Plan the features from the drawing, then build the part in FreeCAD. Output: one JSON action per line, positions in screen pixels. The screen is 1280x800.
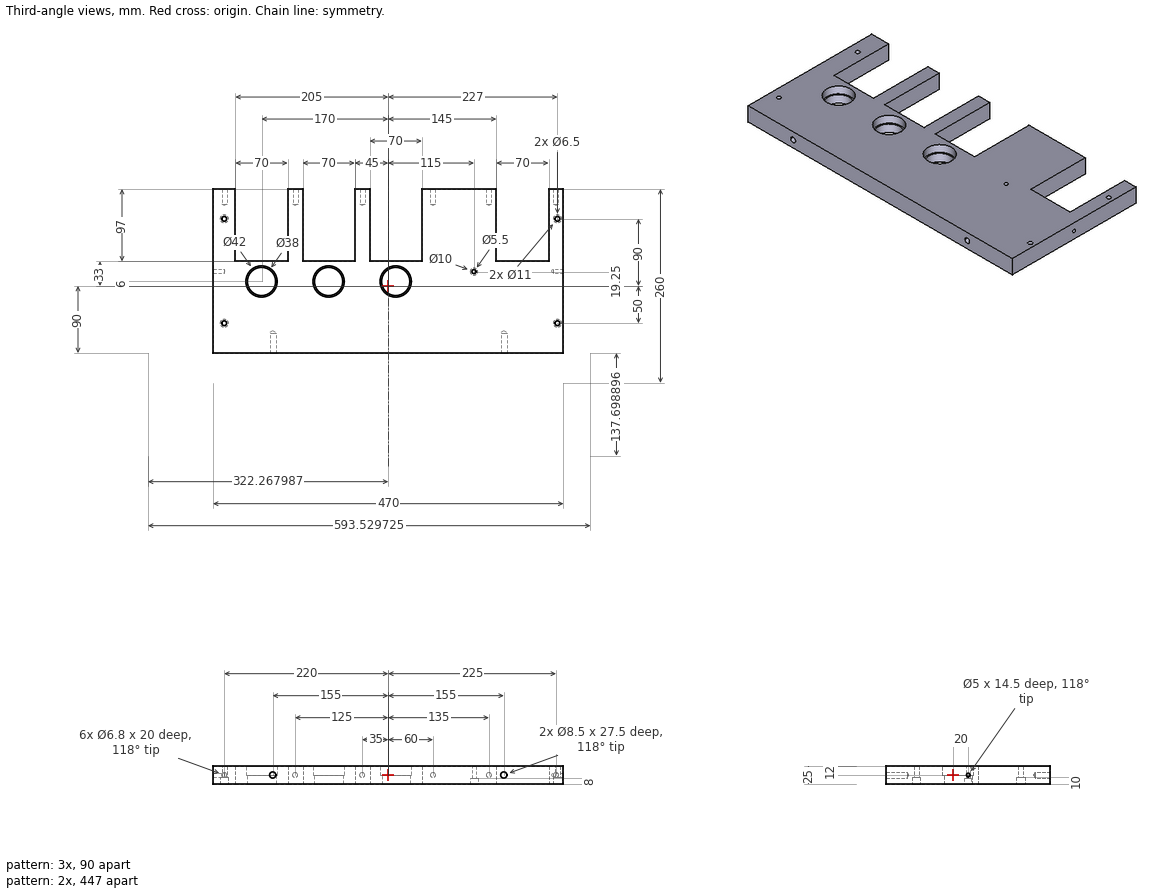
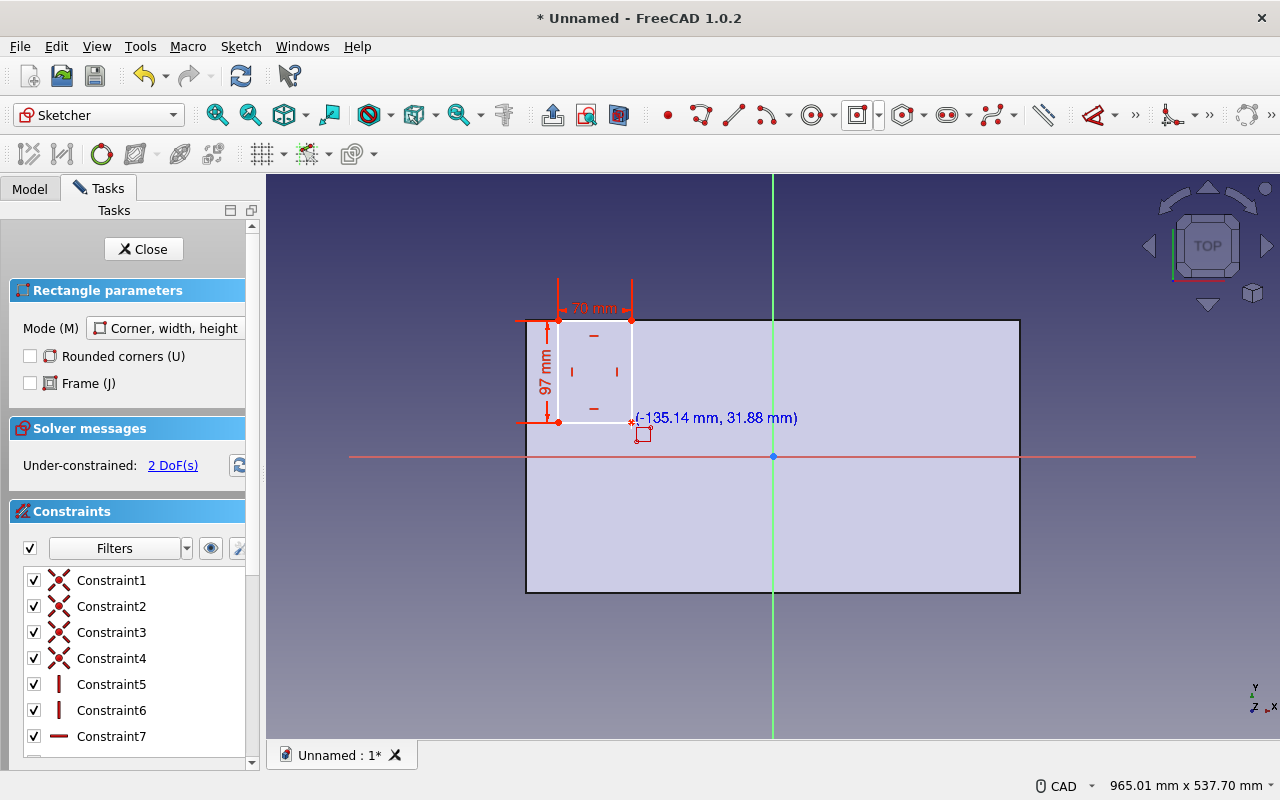
{"action": "left_click", "coordinate": [652, 320]}
{"action": "mouse_move", "coordinate": [726, 422]}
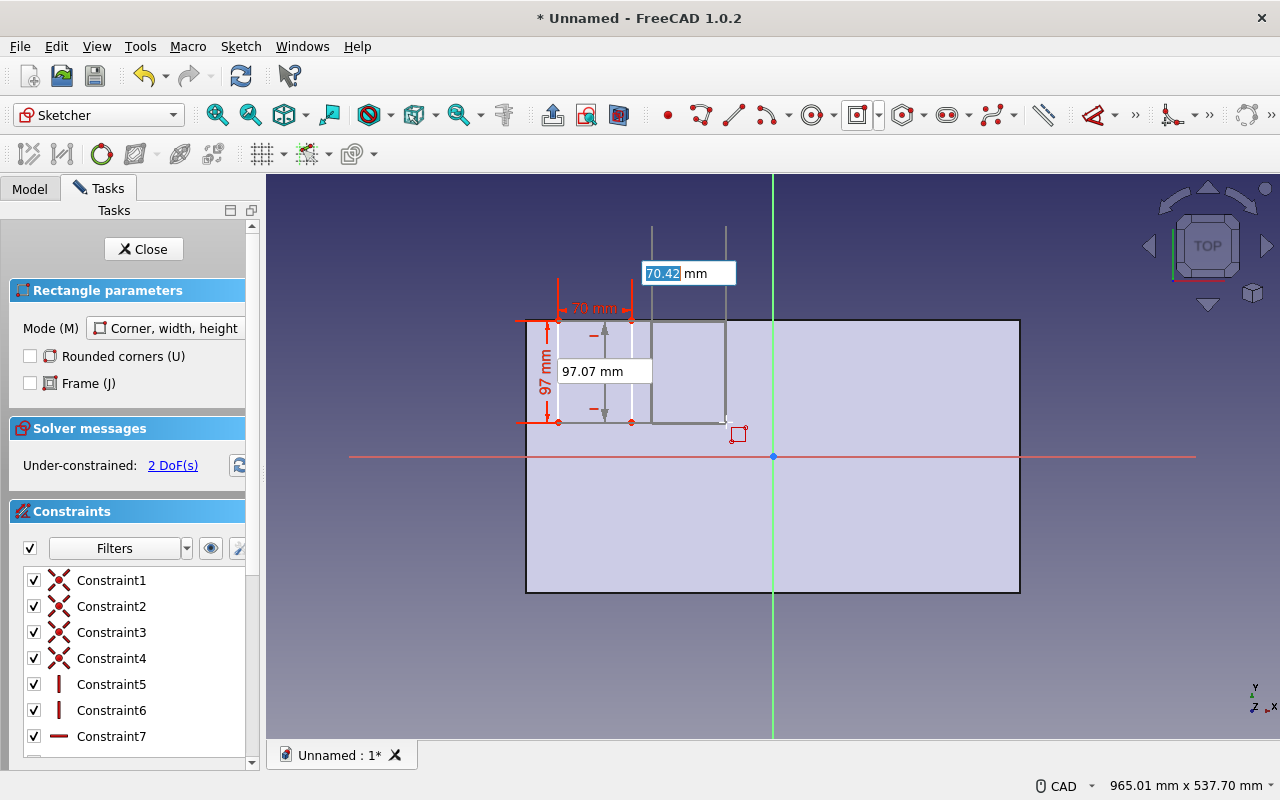
{"action": "type", "text": "70"}
{"action": "key", "text": "Tab"}
{"action": "type", "text": "97"}
{"action": "key", "text": "Return"}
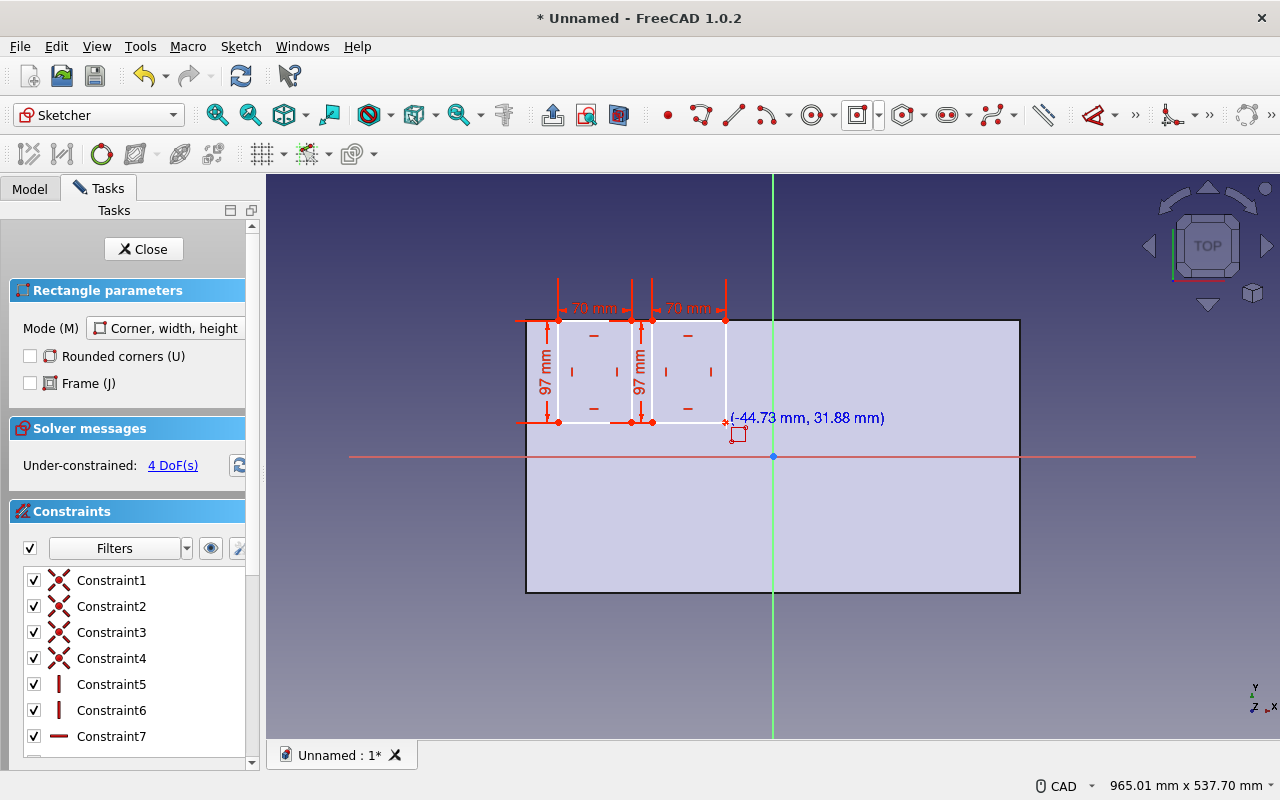
{"action": "left_click", "coordinate": [747, 320]}
{"action": "mouse_move", "coordinate": [820, 422]}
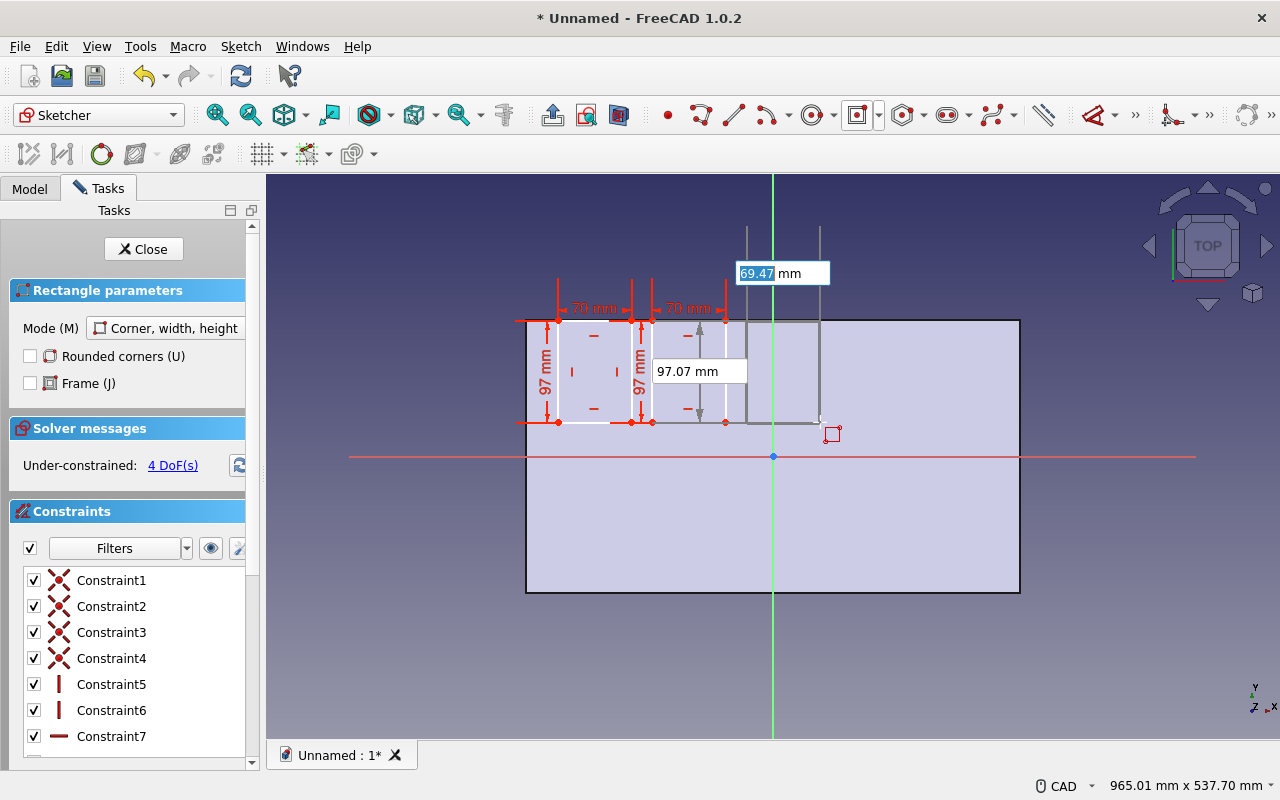
{"action": "type", "text": "70"}
{"action": "key", "text": "Tab"}
{"action": "type", "text": "97"}
{"action": "key", "text": "Return"}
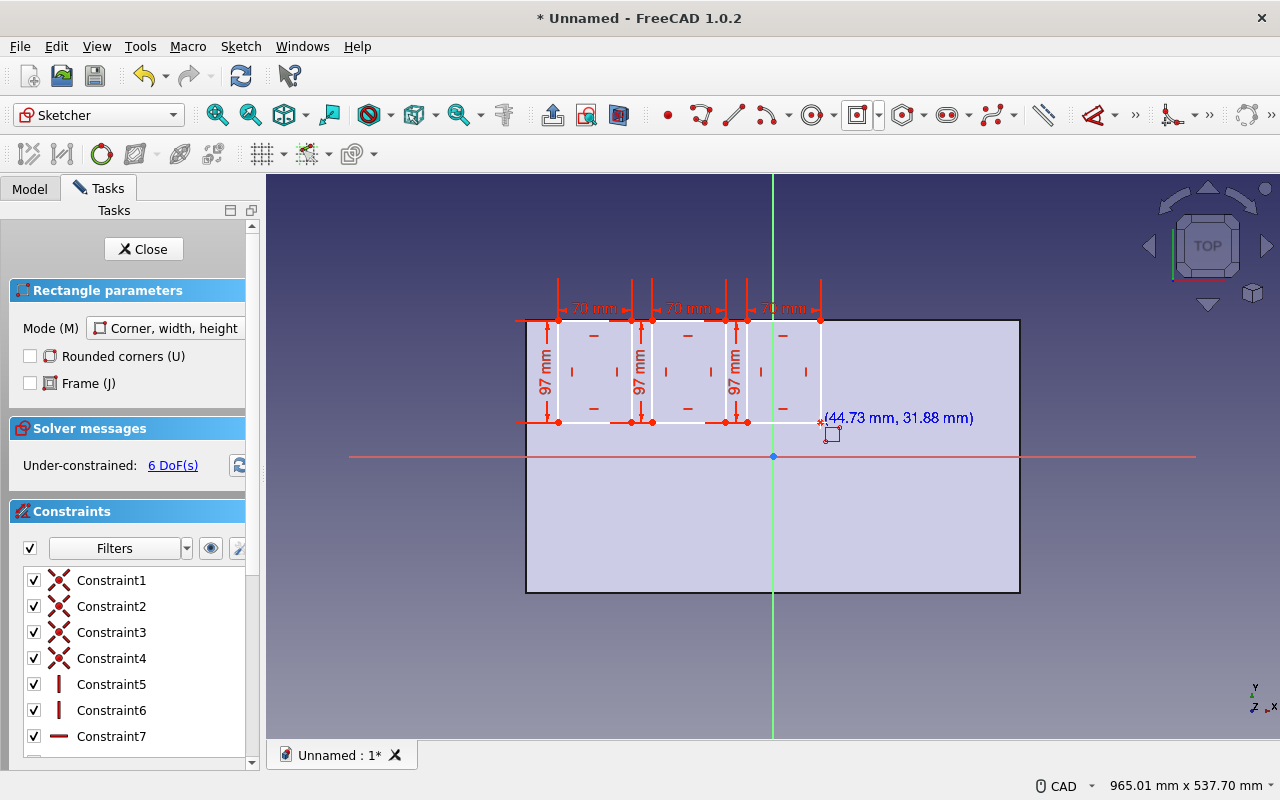
{"action": "left_click", "coordinate": [925, 320]}
{"action": "mouse_move", "coordinate": [999, 422]}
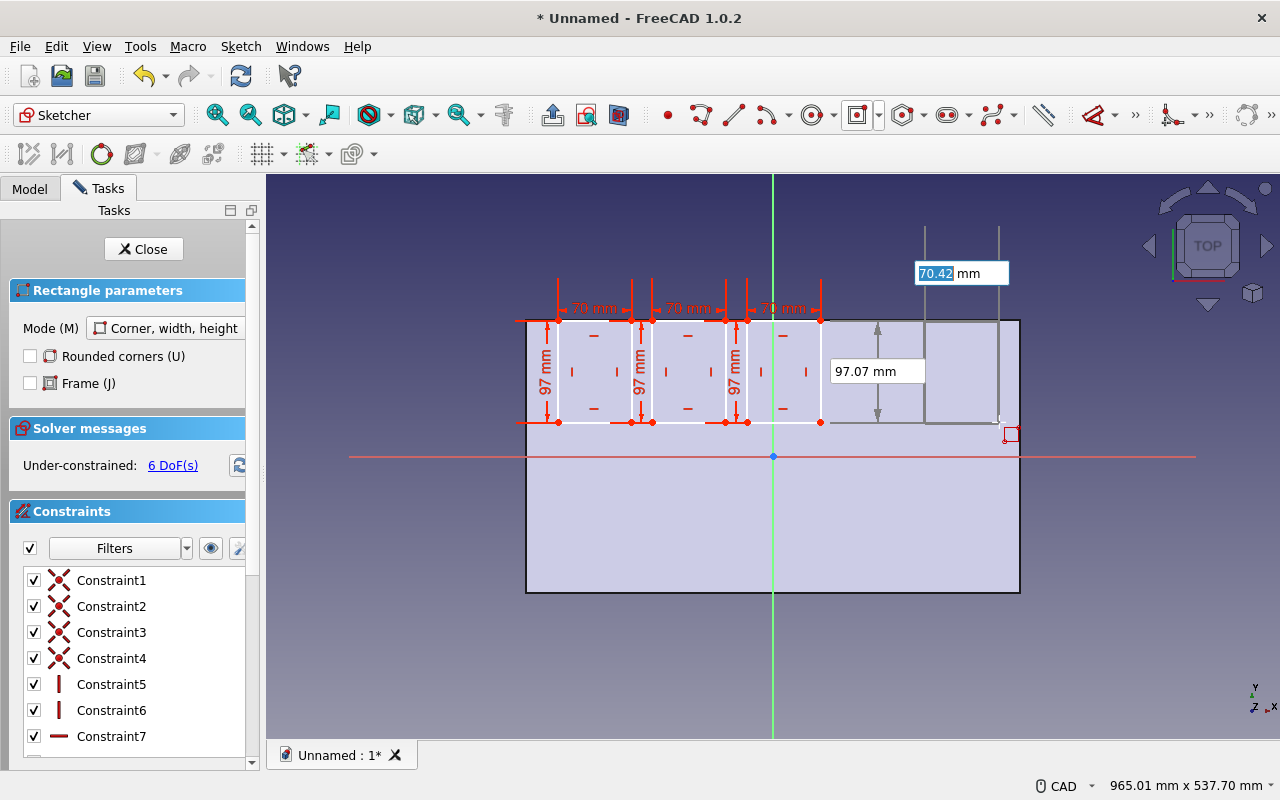
{"action": "type", "text": "70"}
{"action": "key", "text": "Tab"}
{"action": "type", "text": "97"}
{"action": "key", "text": "Return"}
{"action": "key", "text": "Escape"}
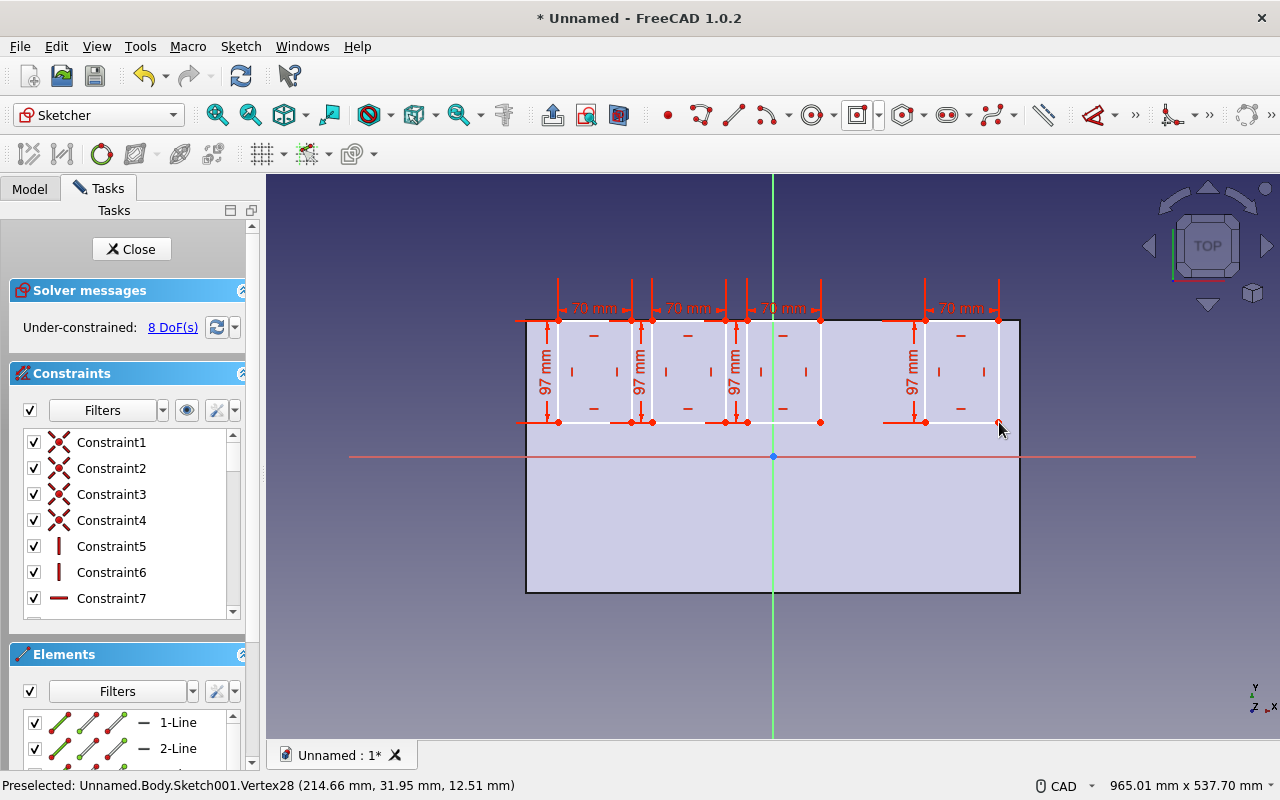
{"action": "left_click", "coordinate": [726, 423]}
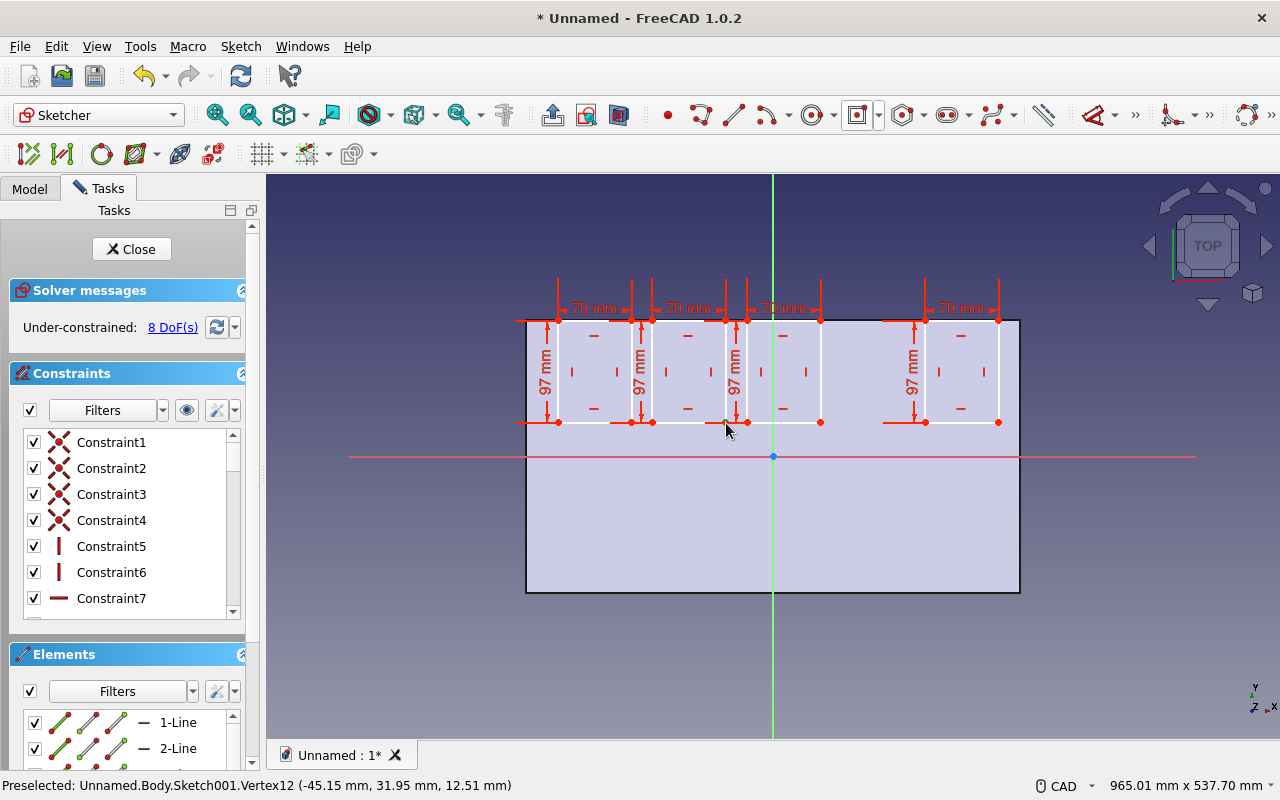
{"action": "left_click", "coordinate": [821, 423]}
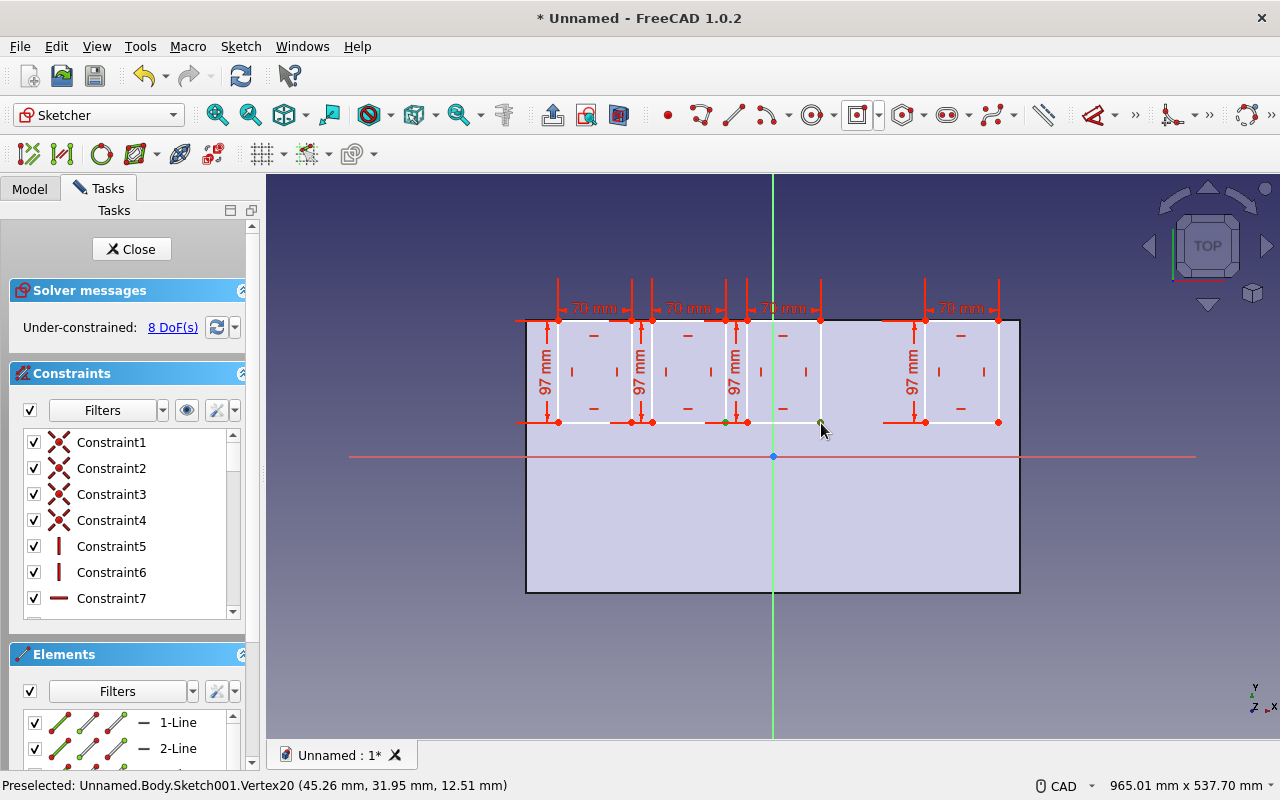
{"action": "left_click", "coordinate": [773, 675]}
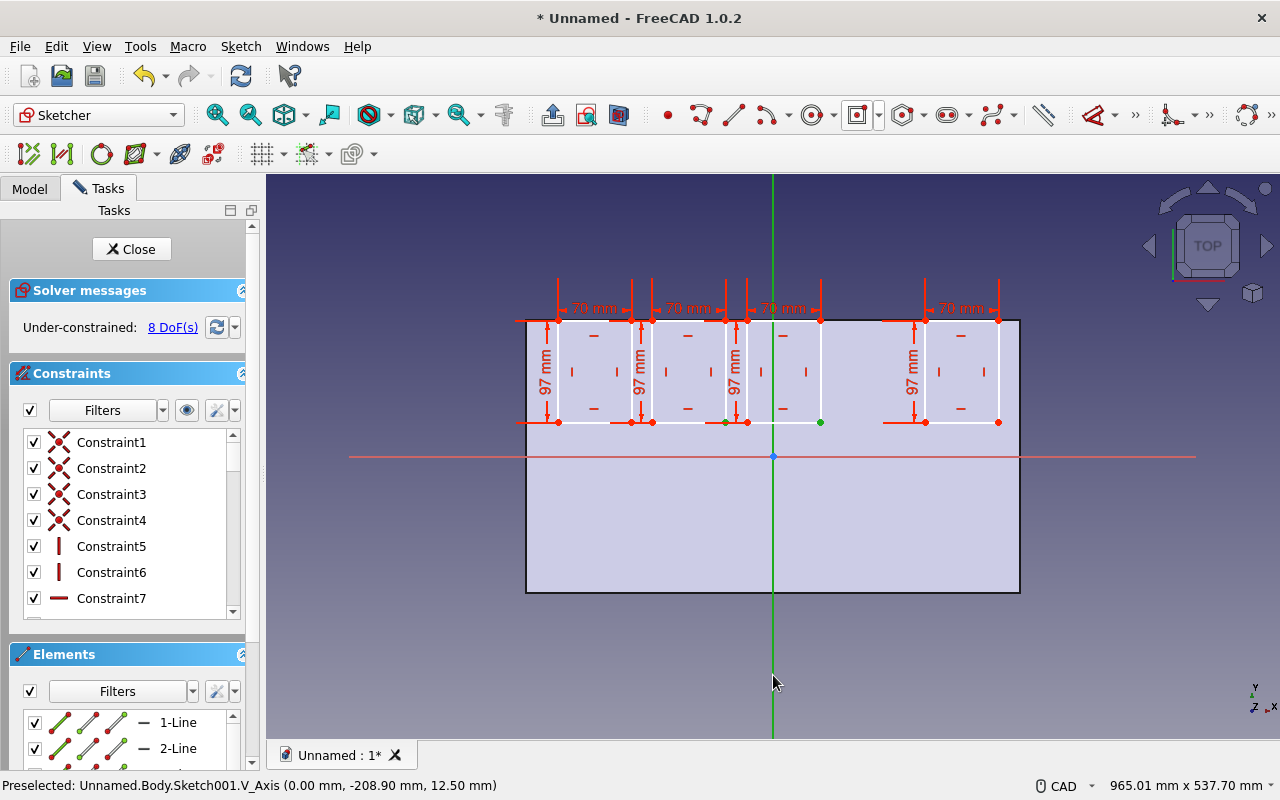
{"action": "key", "text": "s"}